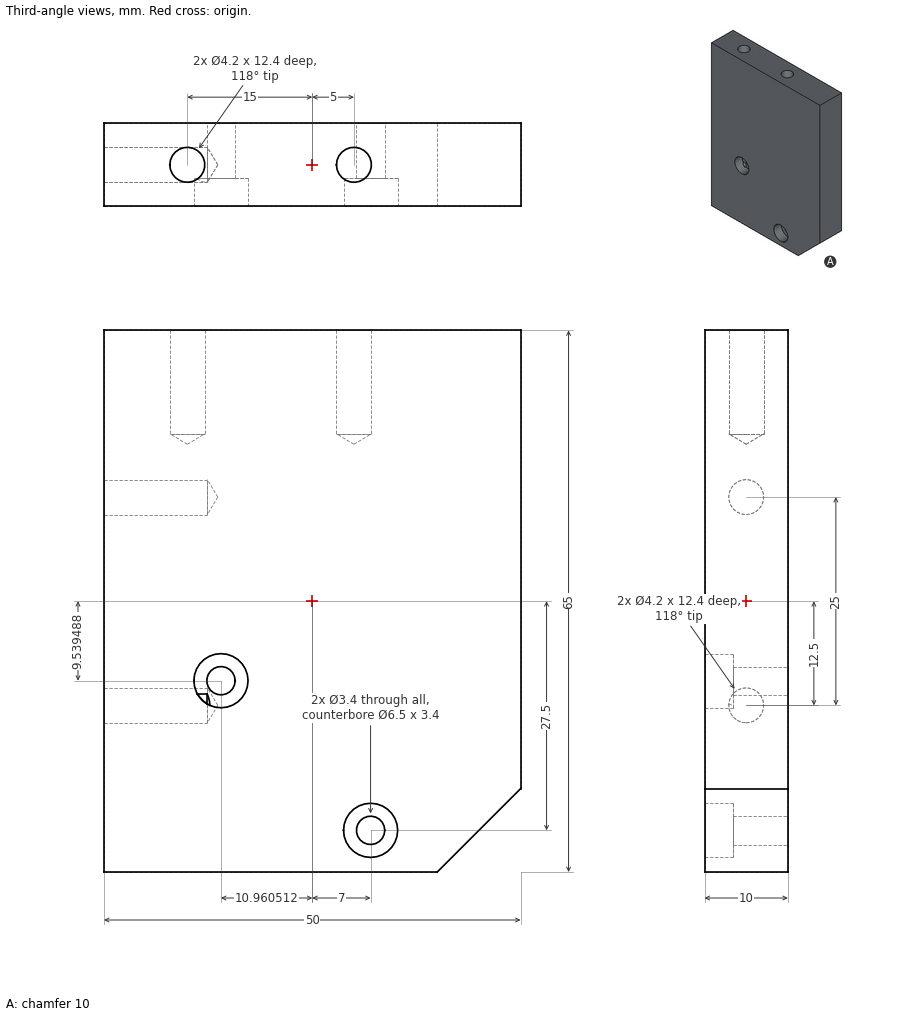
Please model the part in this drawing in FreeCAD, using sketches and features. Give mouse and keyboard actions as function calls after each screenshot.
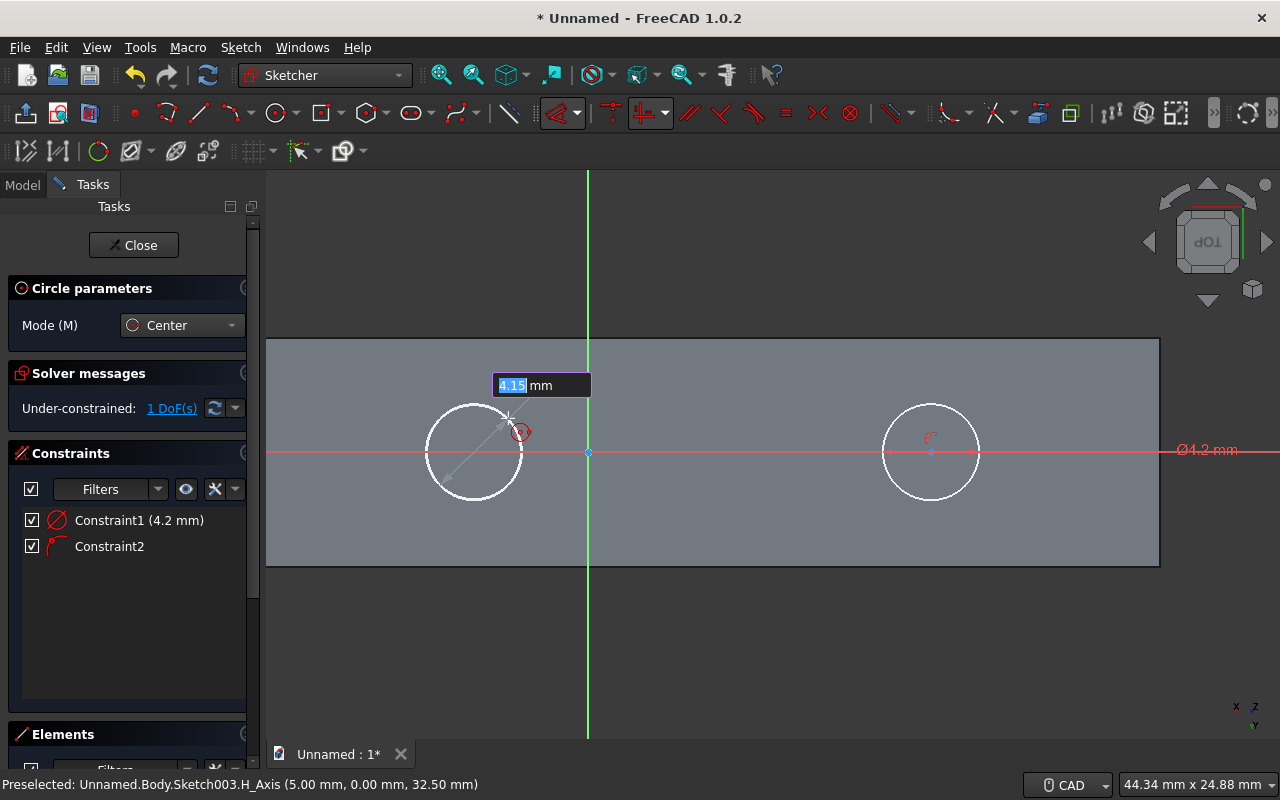
text(4.2)
key(Return)
key(Escape)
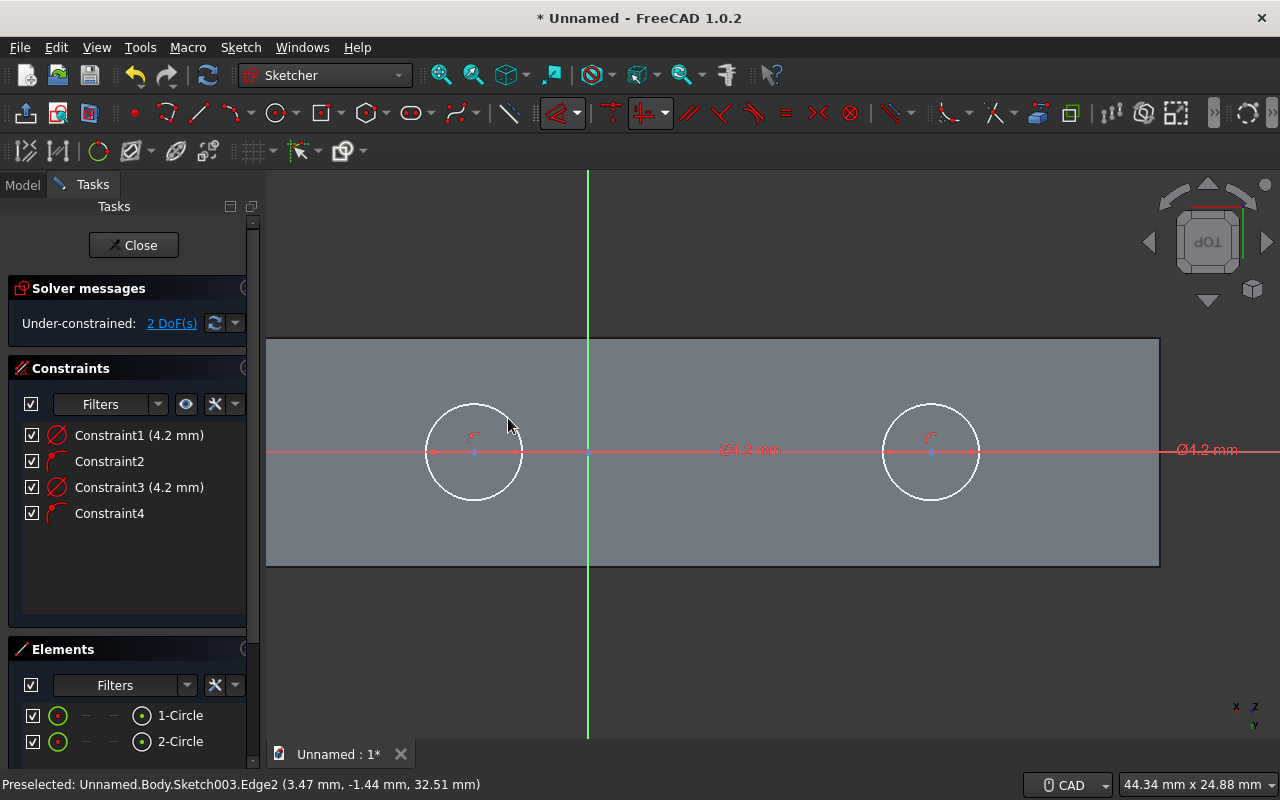
key(d)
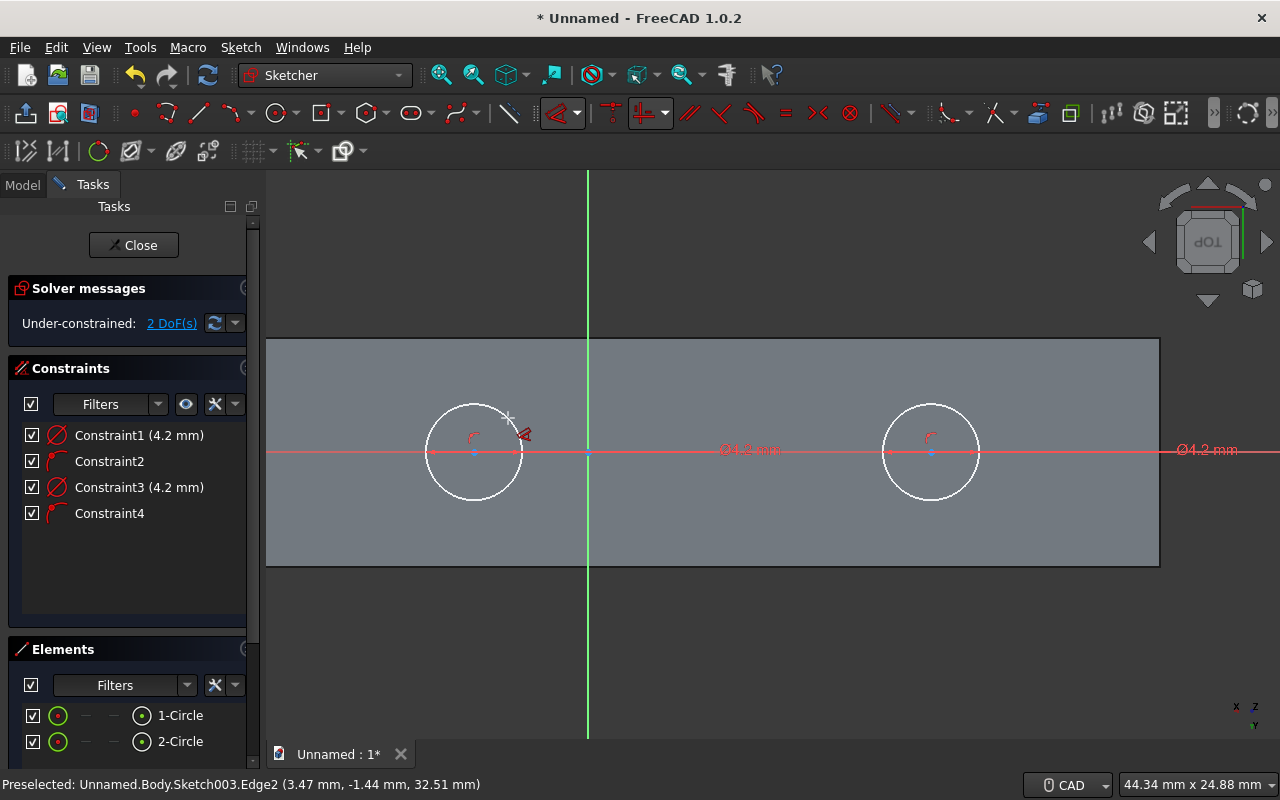
click(474, 452)
click(531, 486)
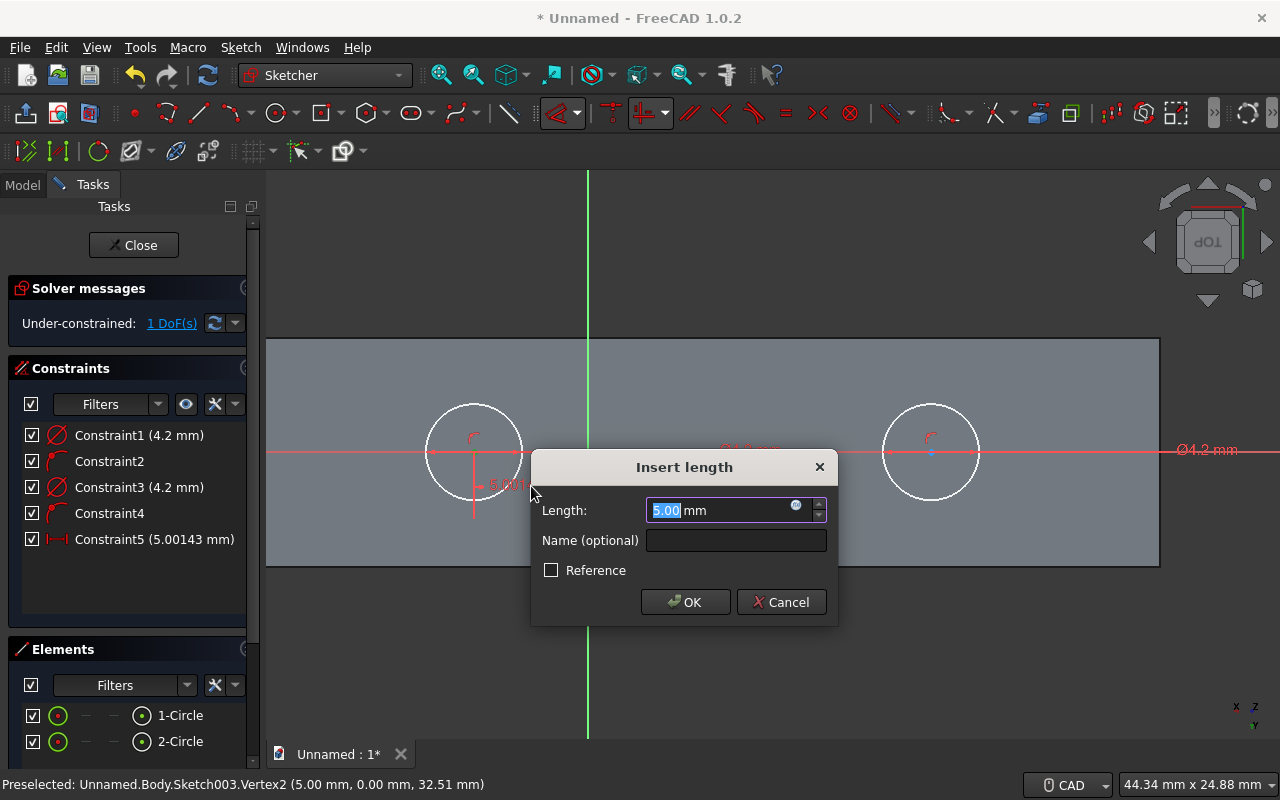
text(5)
key(Return)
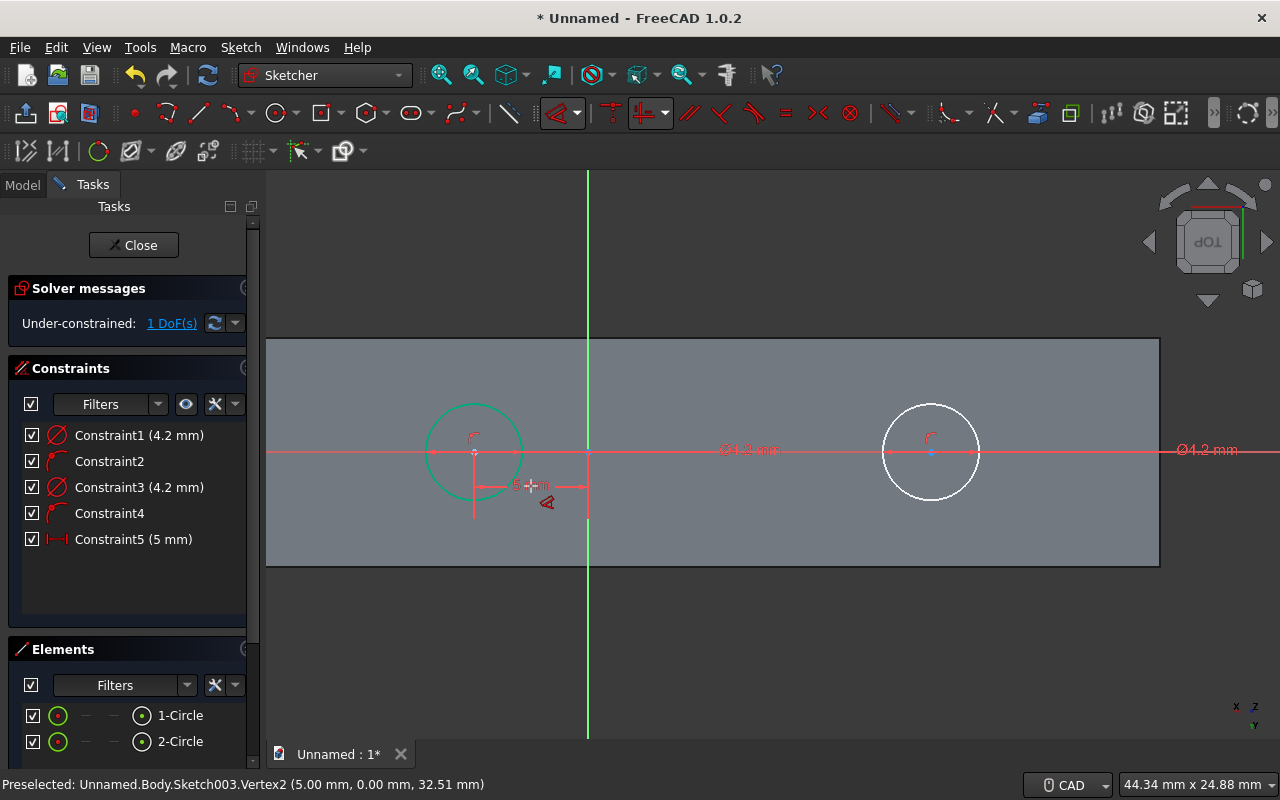
click(931, 452)
click(760, 486)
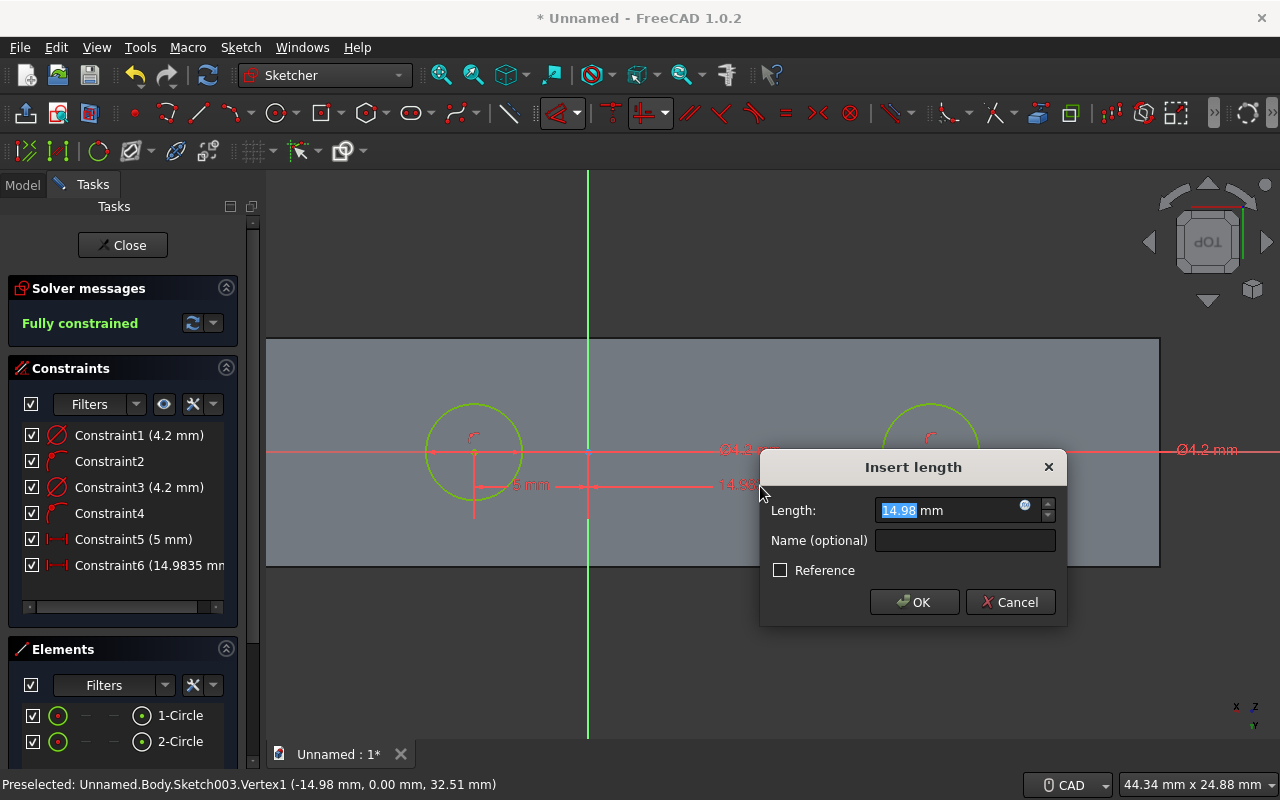
text(15)
key(Return)
key(Escape)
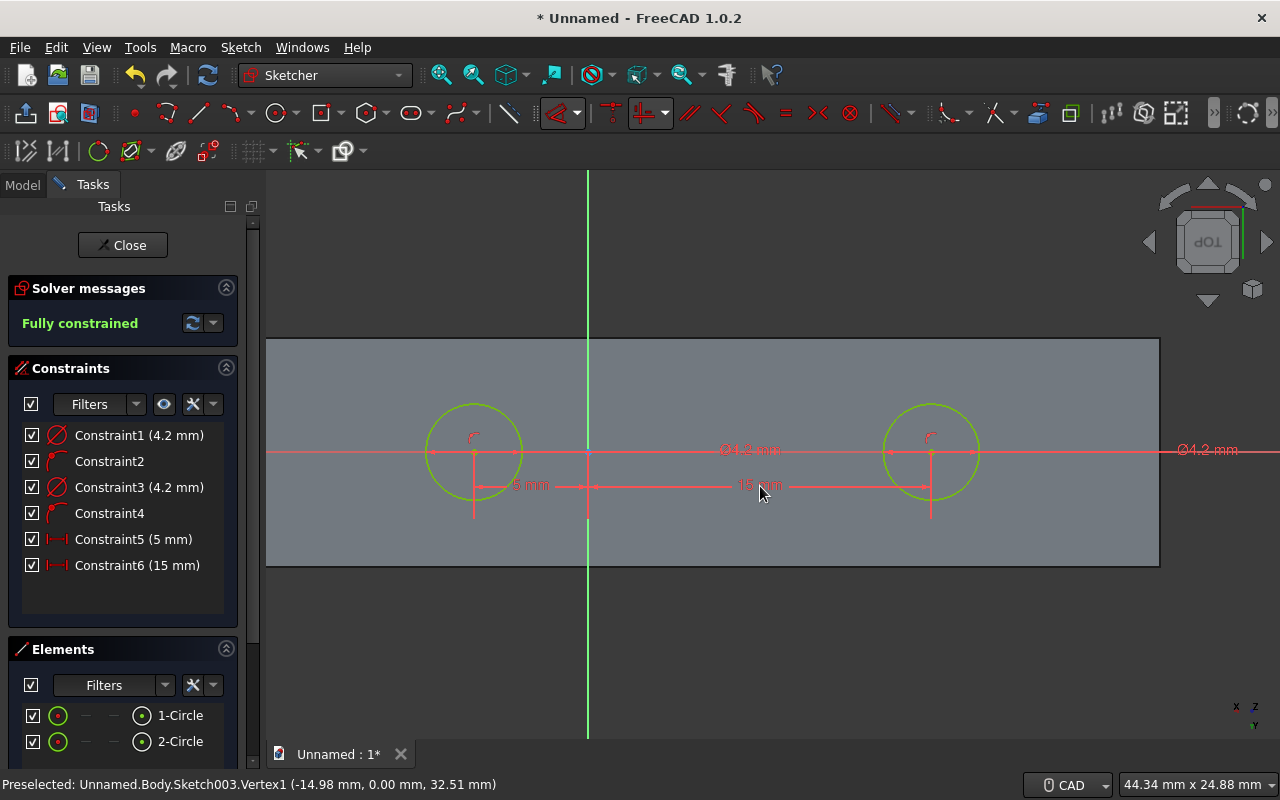
click(123, 245)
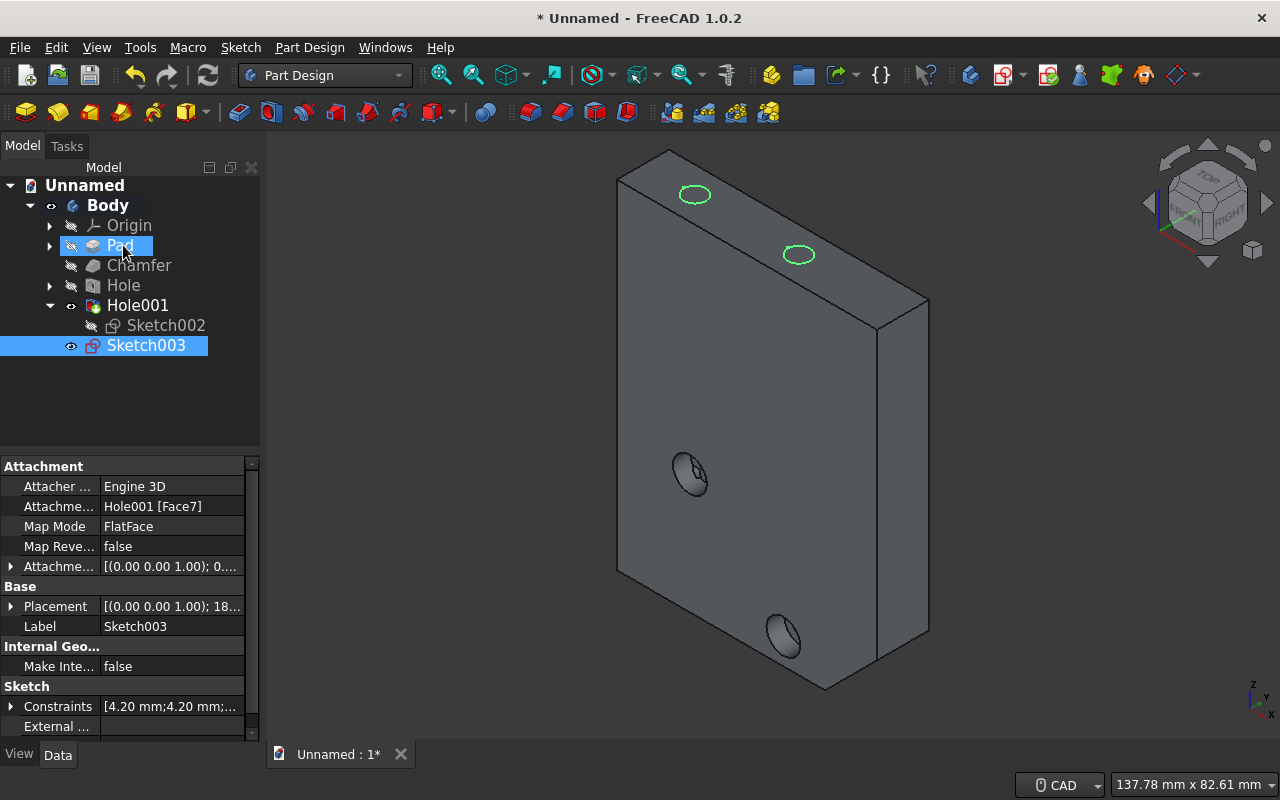
click(272, 112)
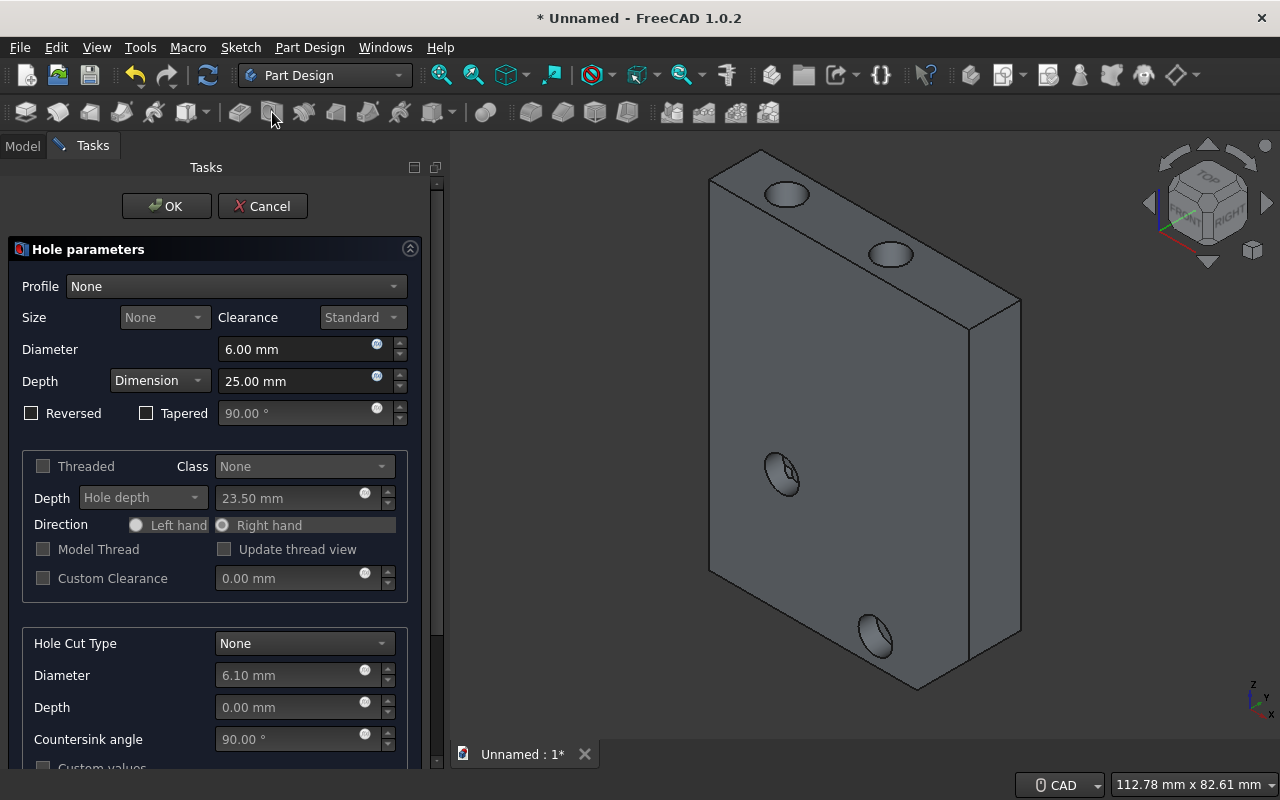
triple_click(305, 349)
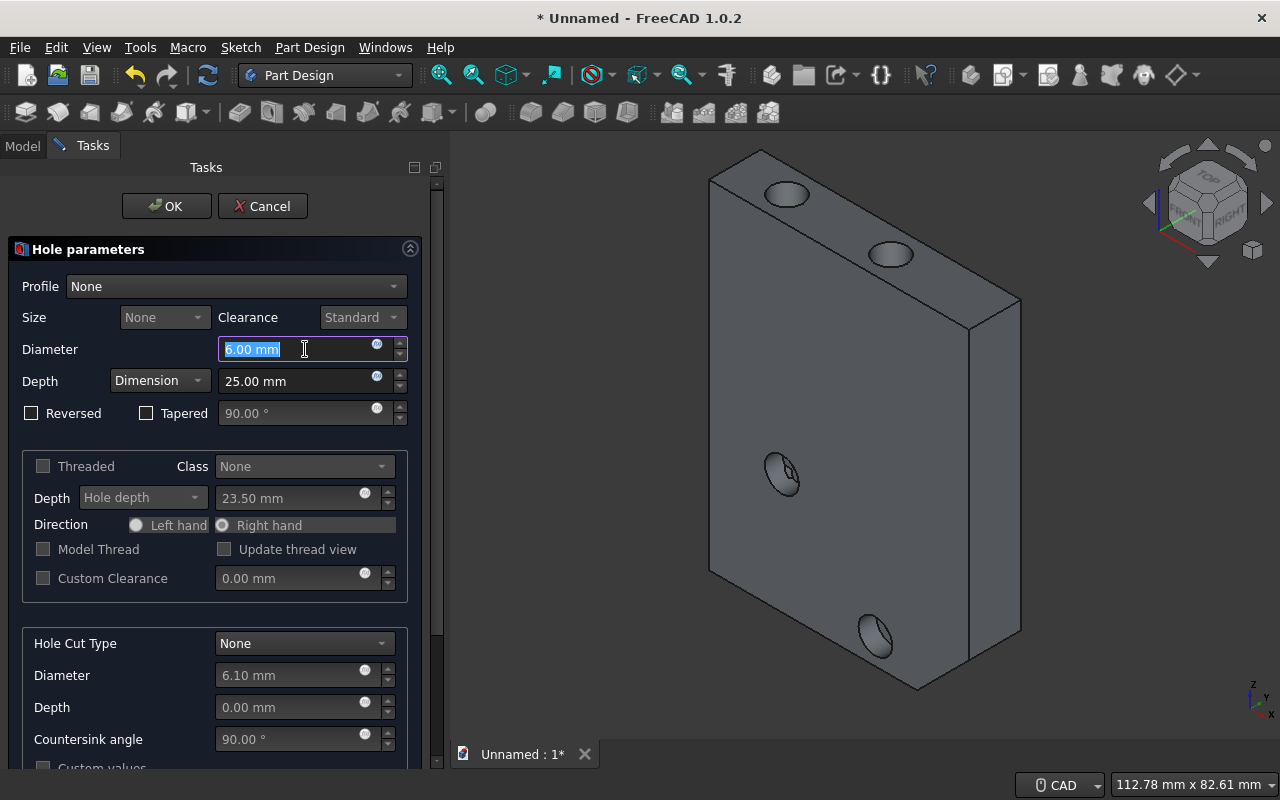
text(4.2)
key(Tab)